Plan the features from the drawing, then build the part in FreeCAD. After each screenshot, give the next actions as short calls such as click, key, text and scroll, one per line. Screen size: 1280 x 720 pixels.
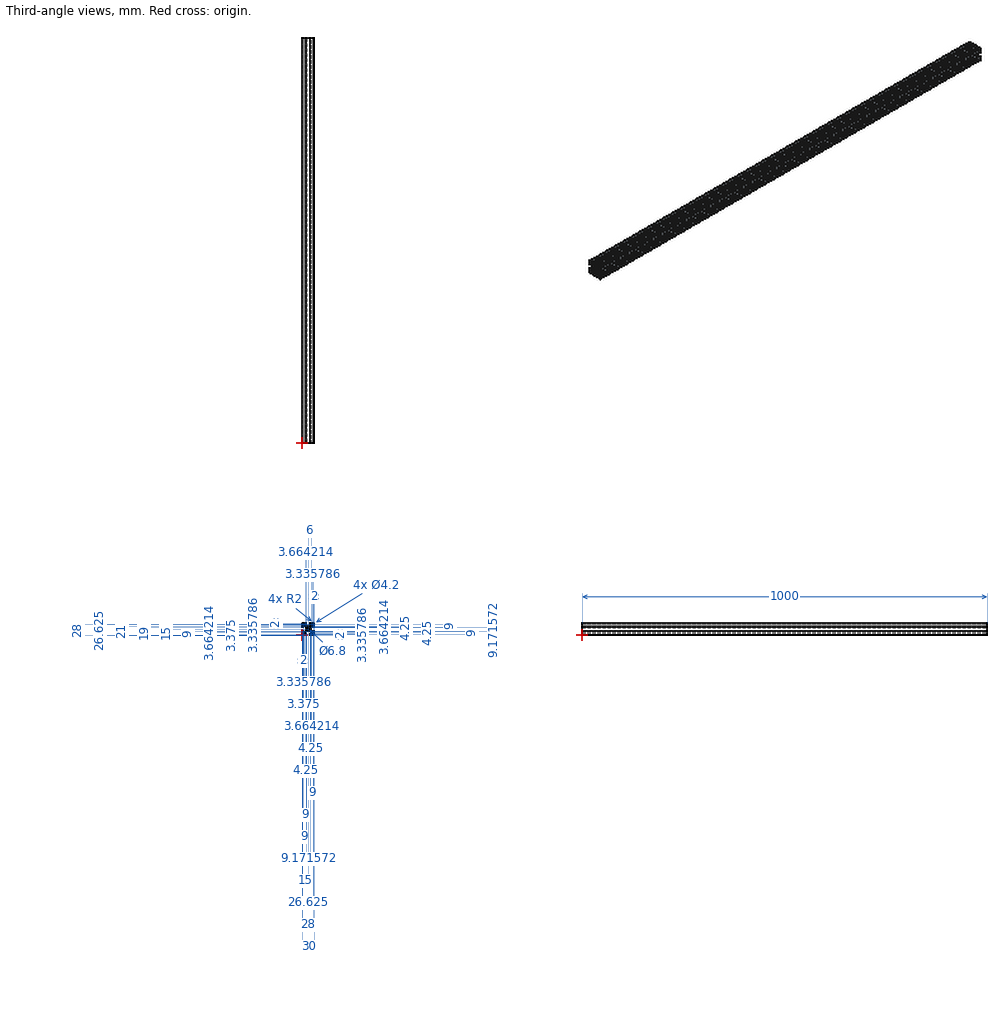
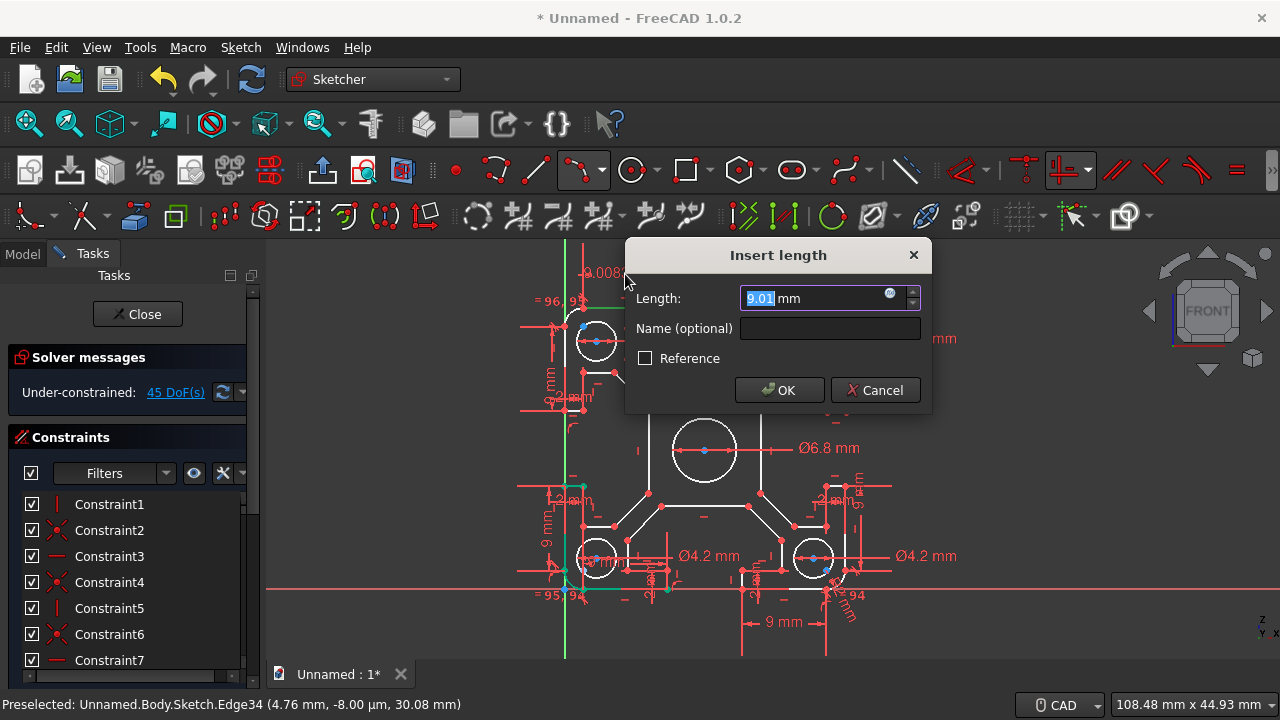
text(9)
key(Return)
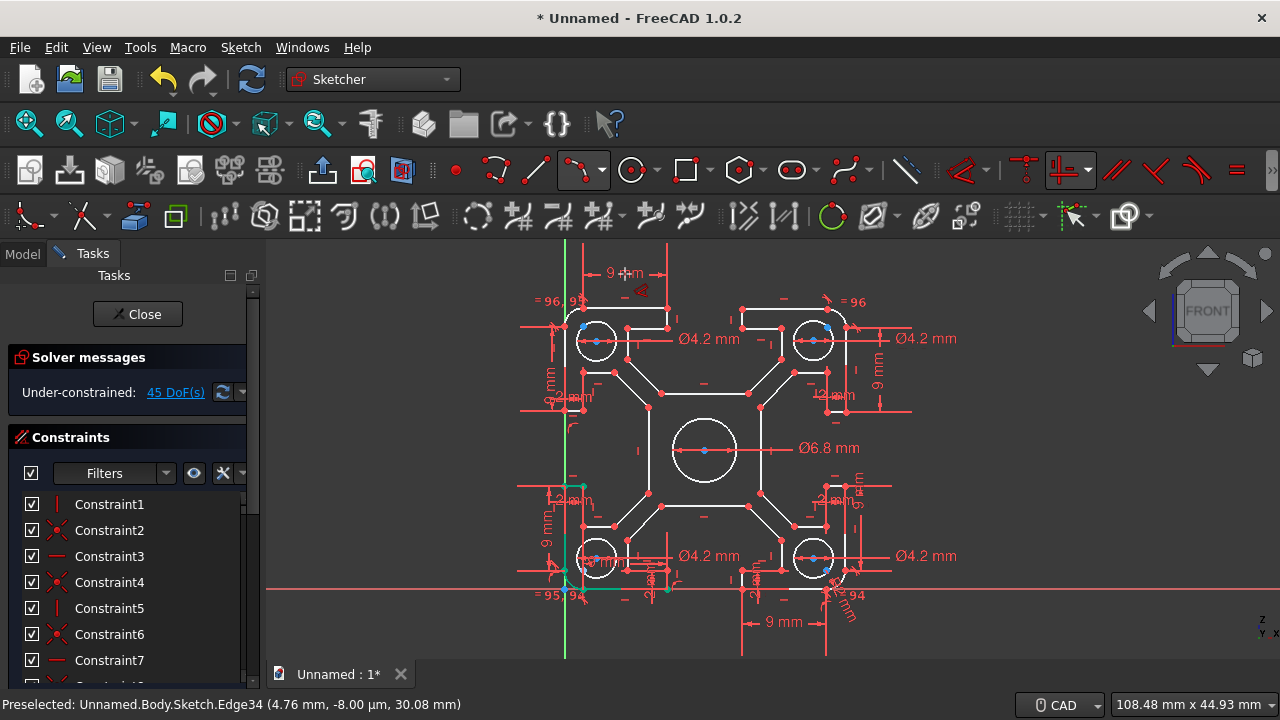
scroll(667, 318, up, 4)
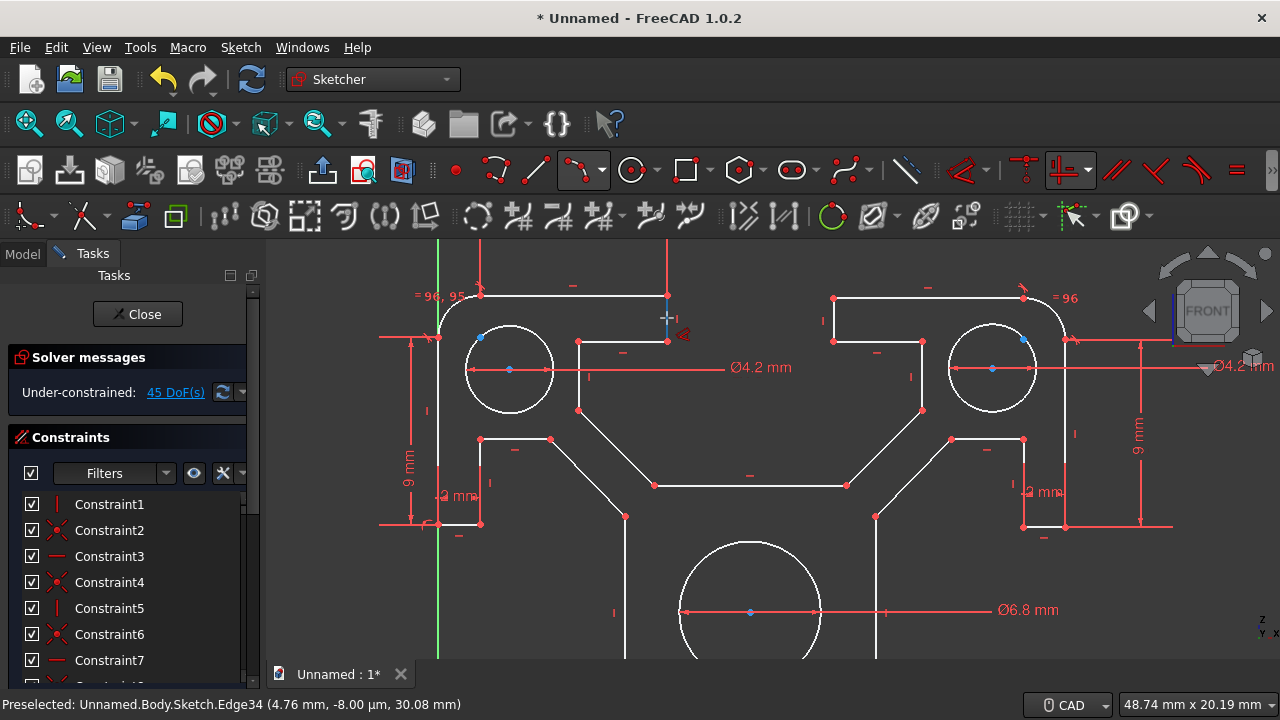
click(667, 319)
click(633, 319)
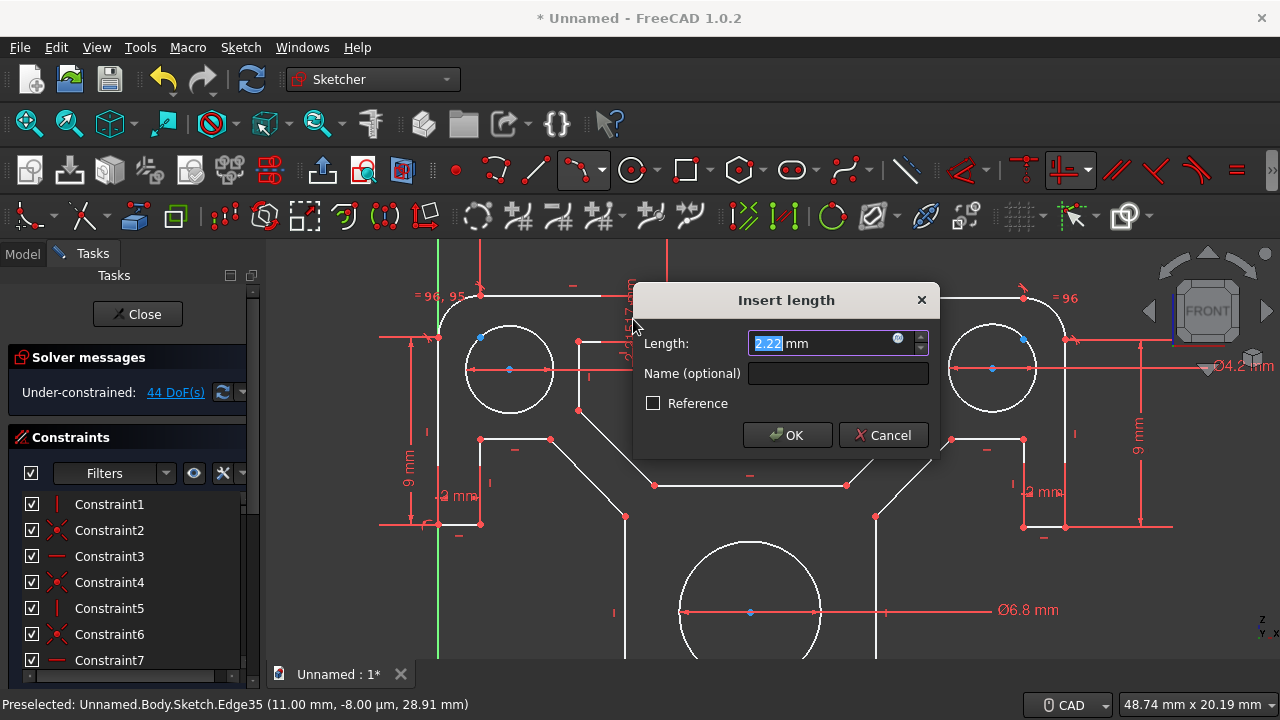
text(2)
key(Return)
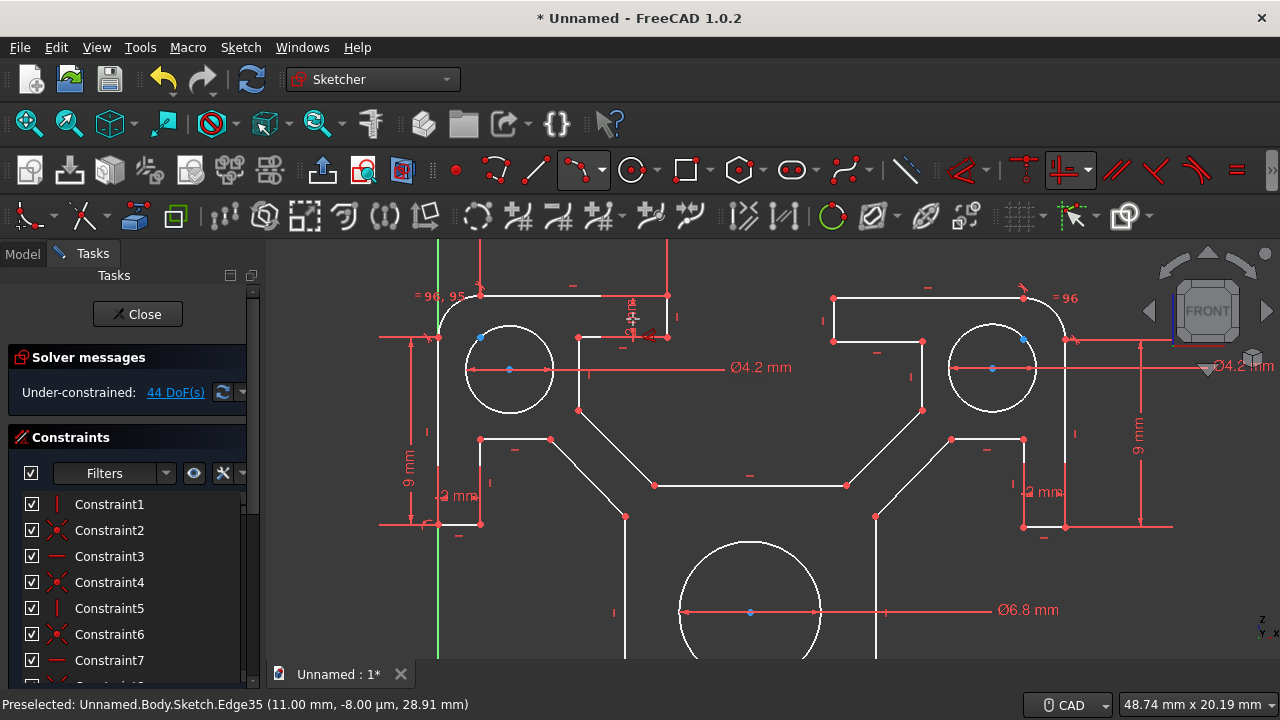
click(834, 329)
click(868, 320)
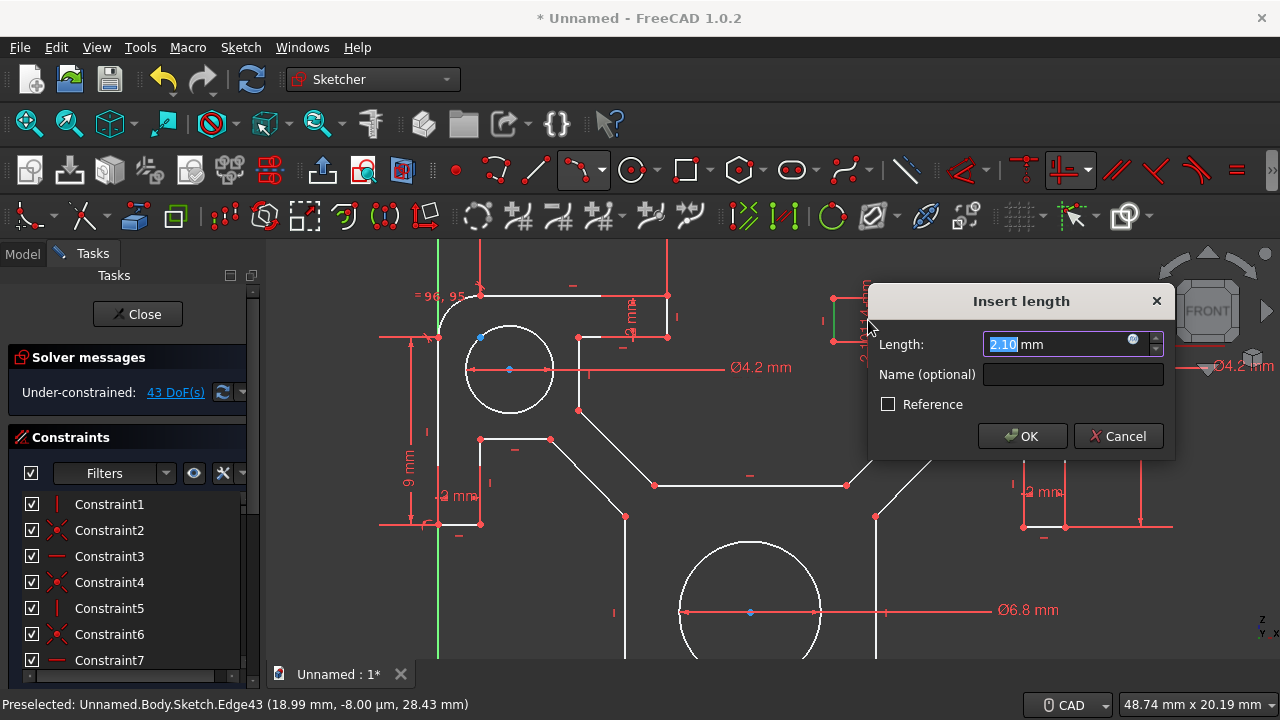
text(2)
key(Return)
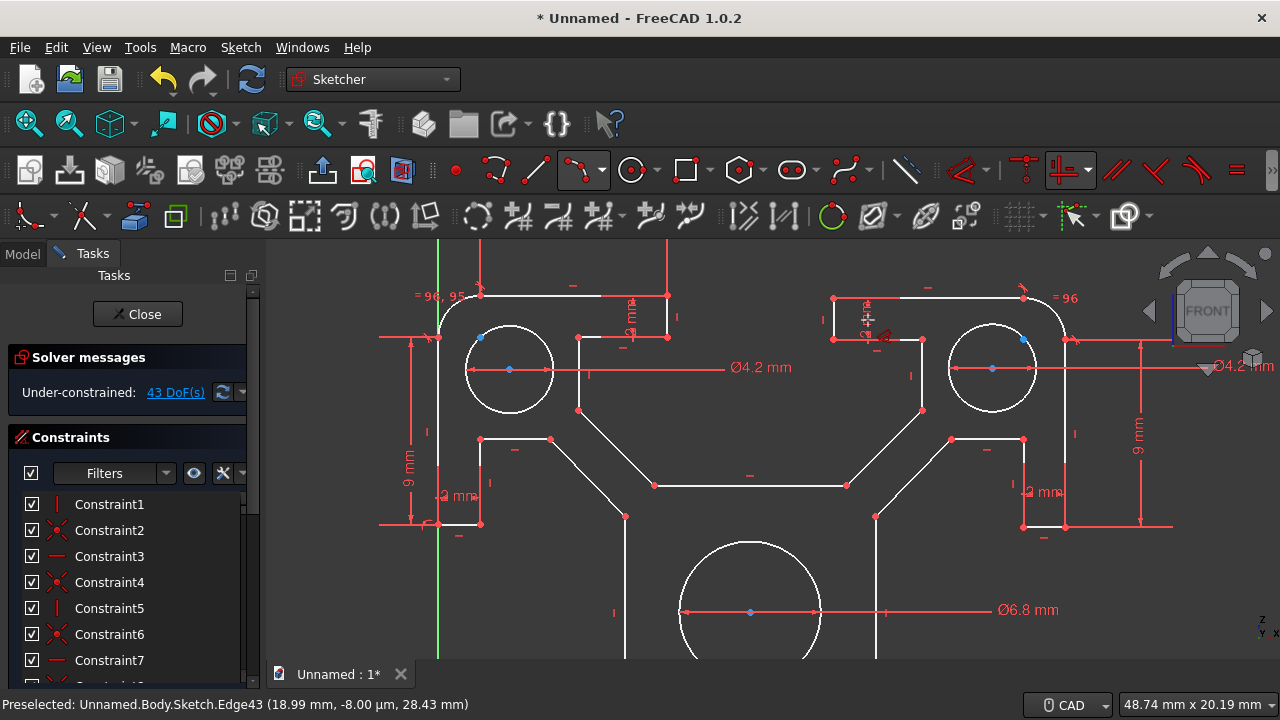
click(891, 298)
click(885, 356)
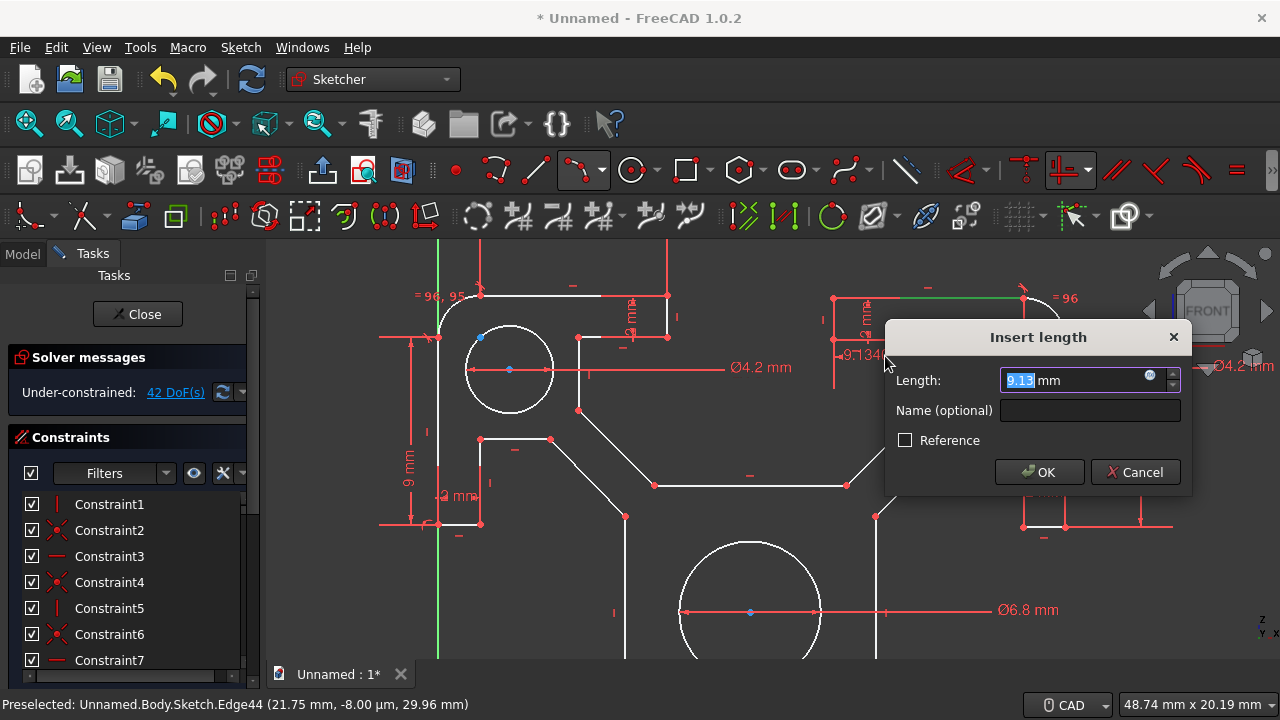
text(9)
key(Return)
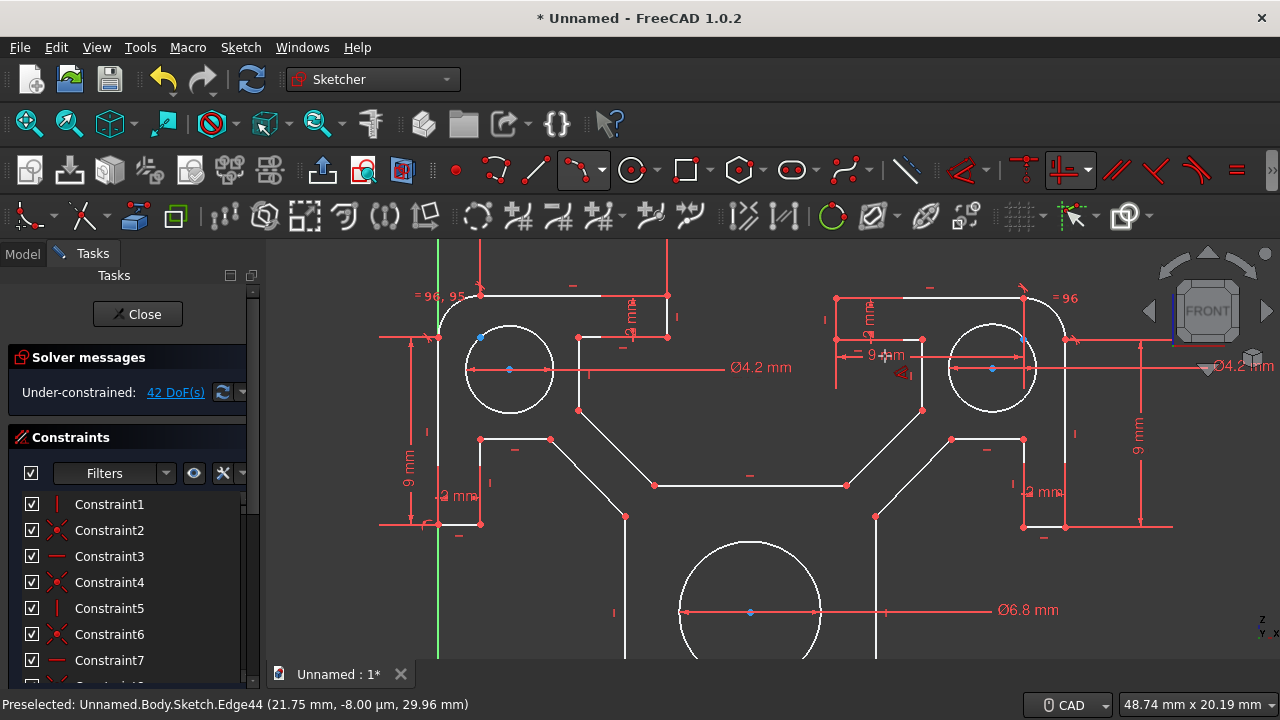
scroll(667, 318, down, 4)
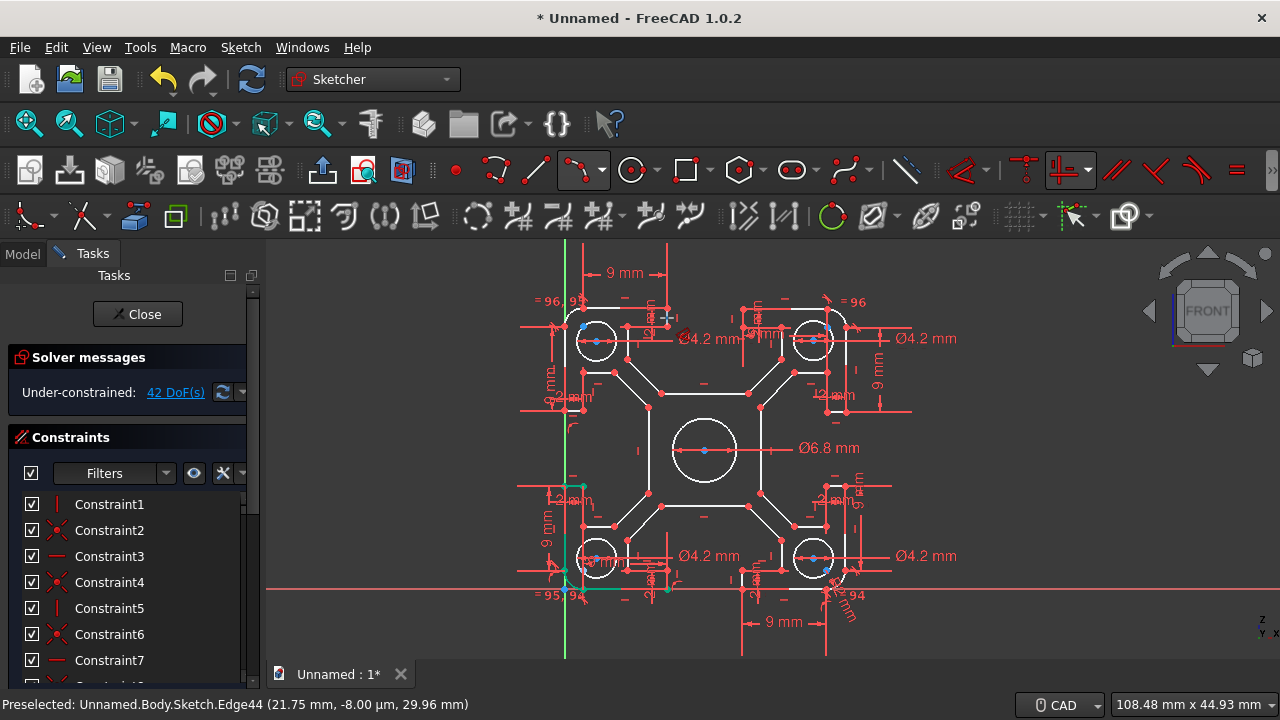
click(748, 506)
click(531, 567)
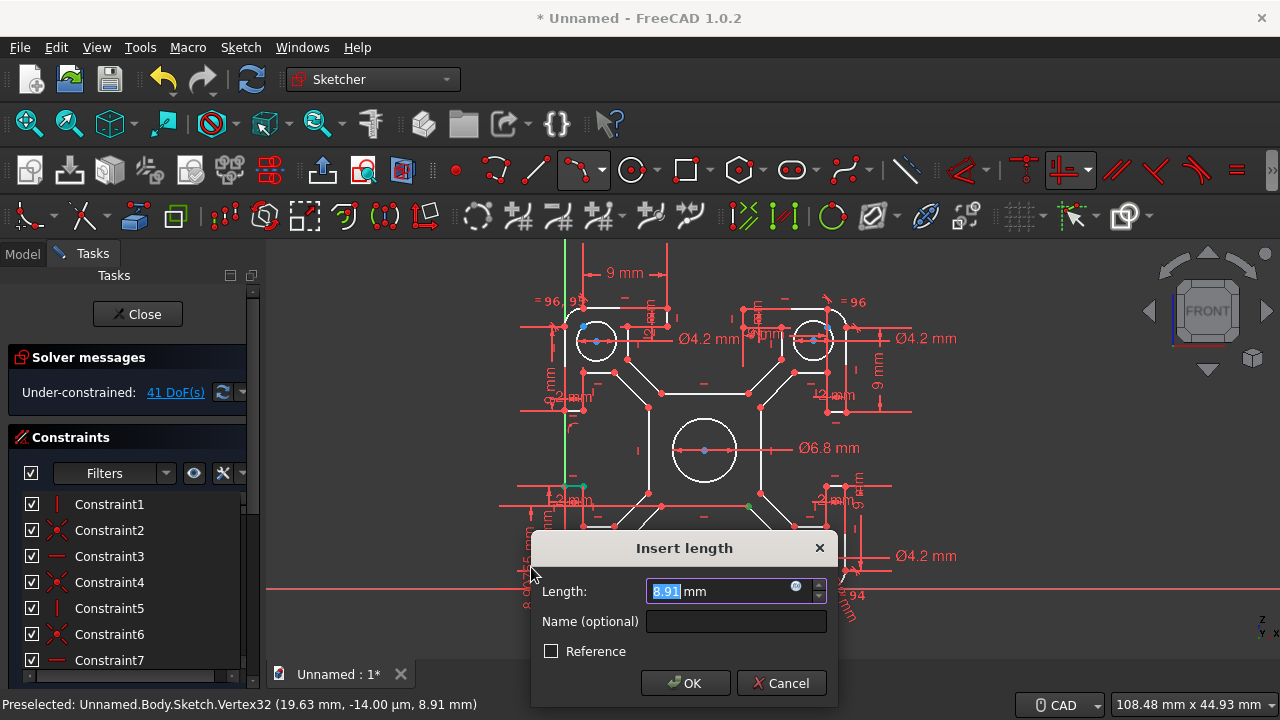
text(9)
key(Return)